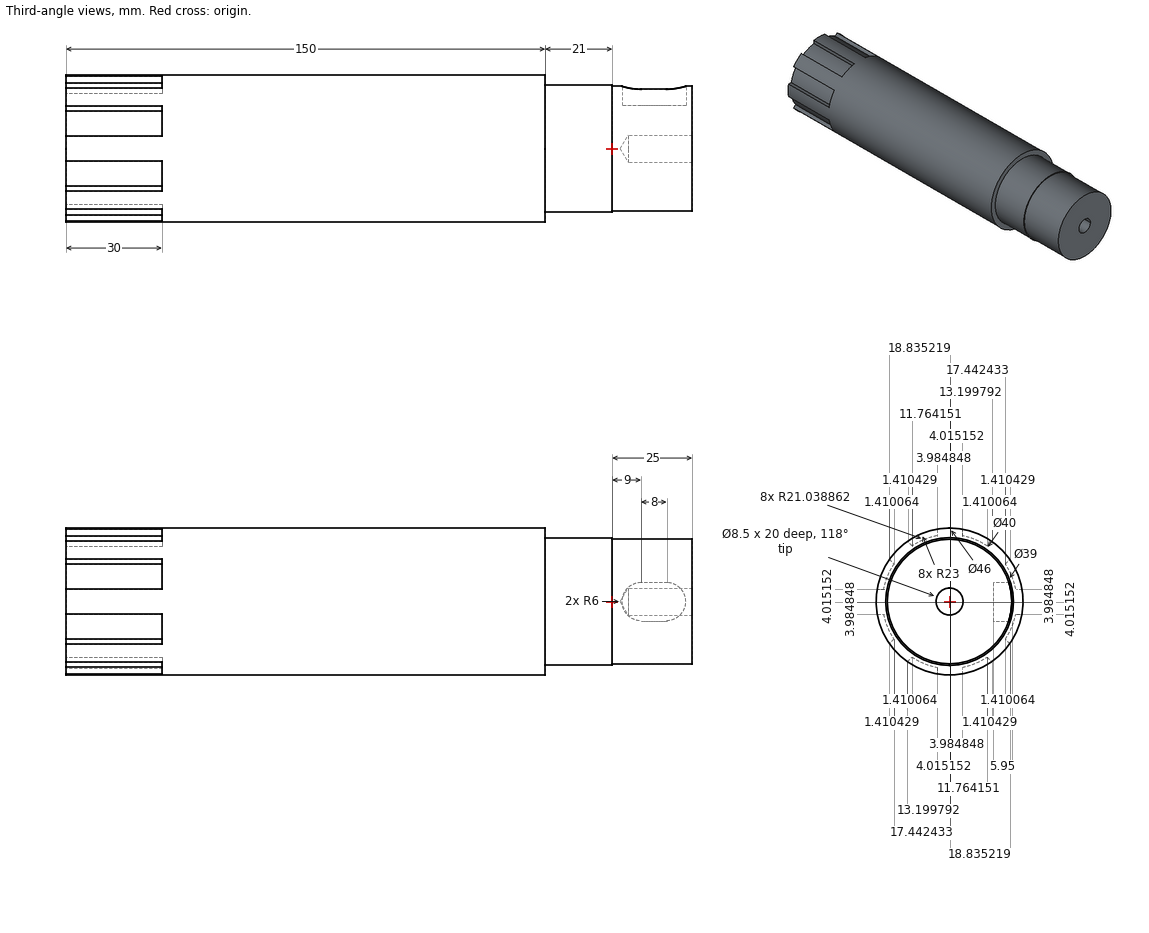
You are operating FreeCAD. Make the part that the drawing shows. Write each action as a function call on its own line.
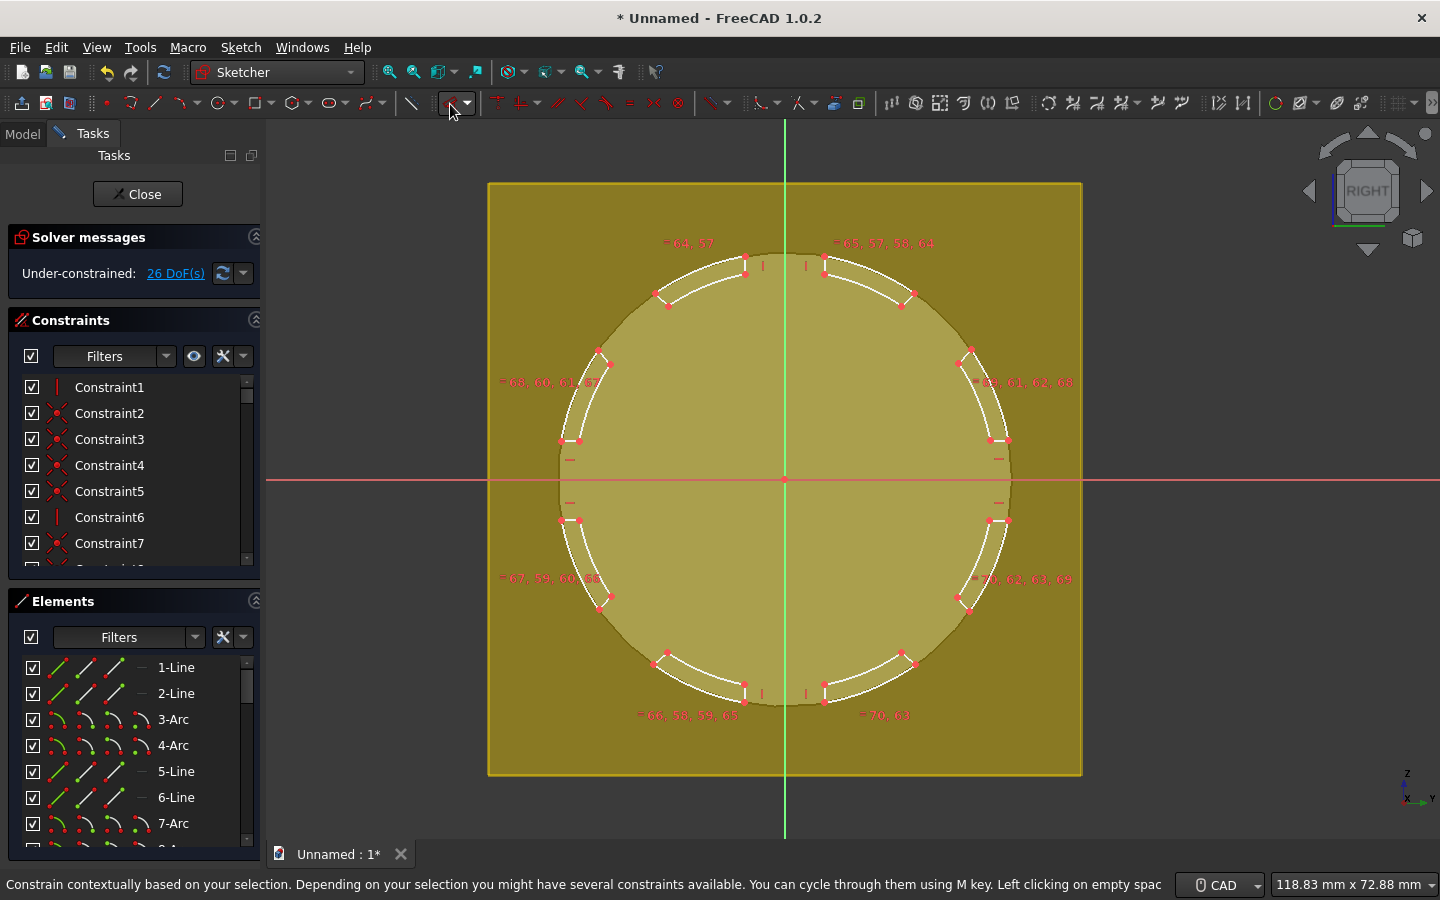
click(721, 280)
click(711, 250)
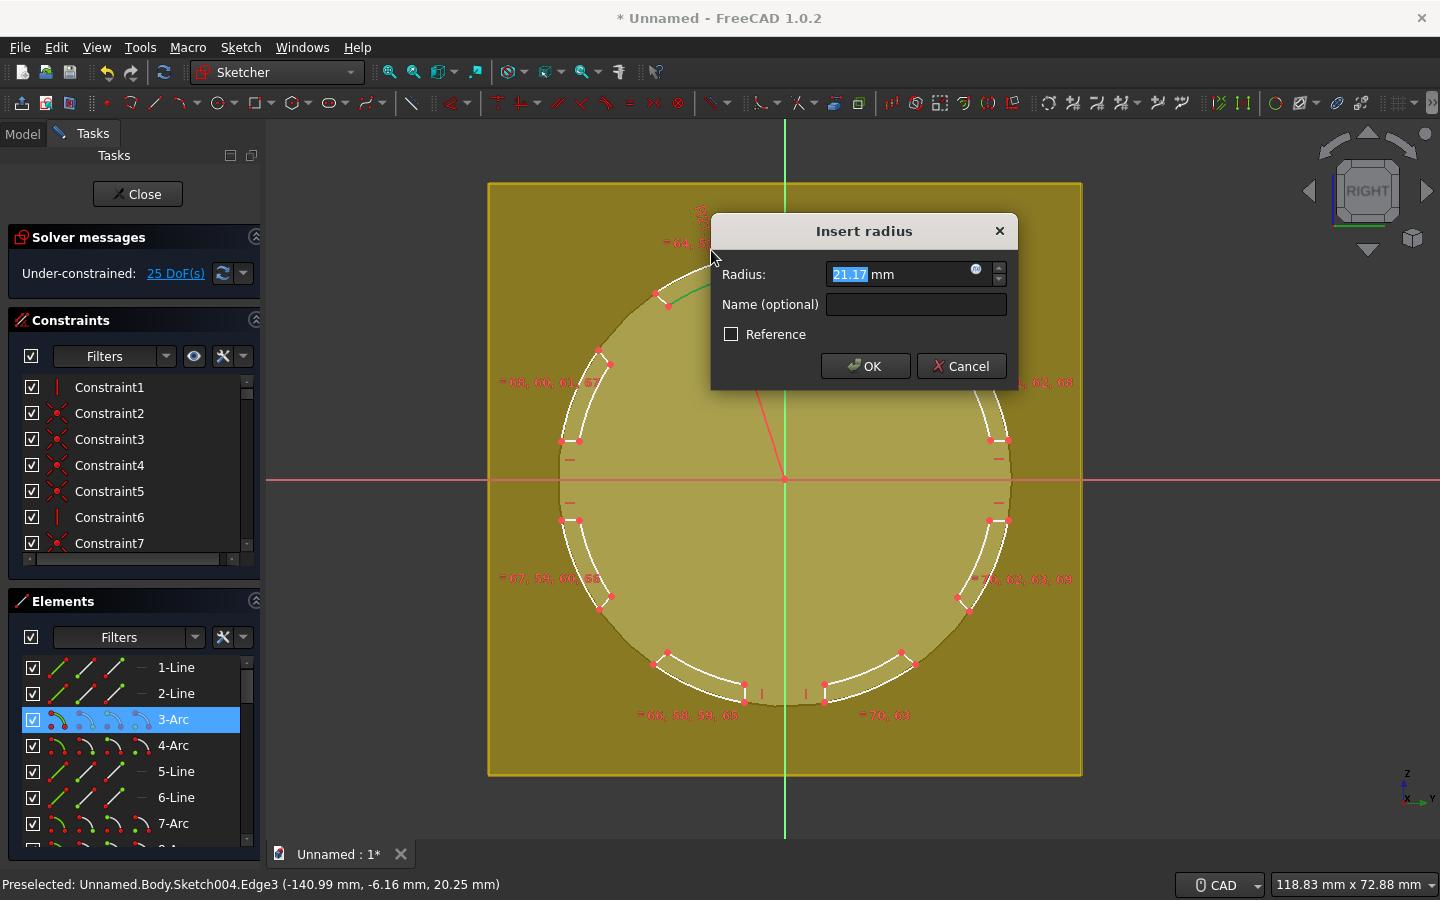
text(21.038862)
key(Return)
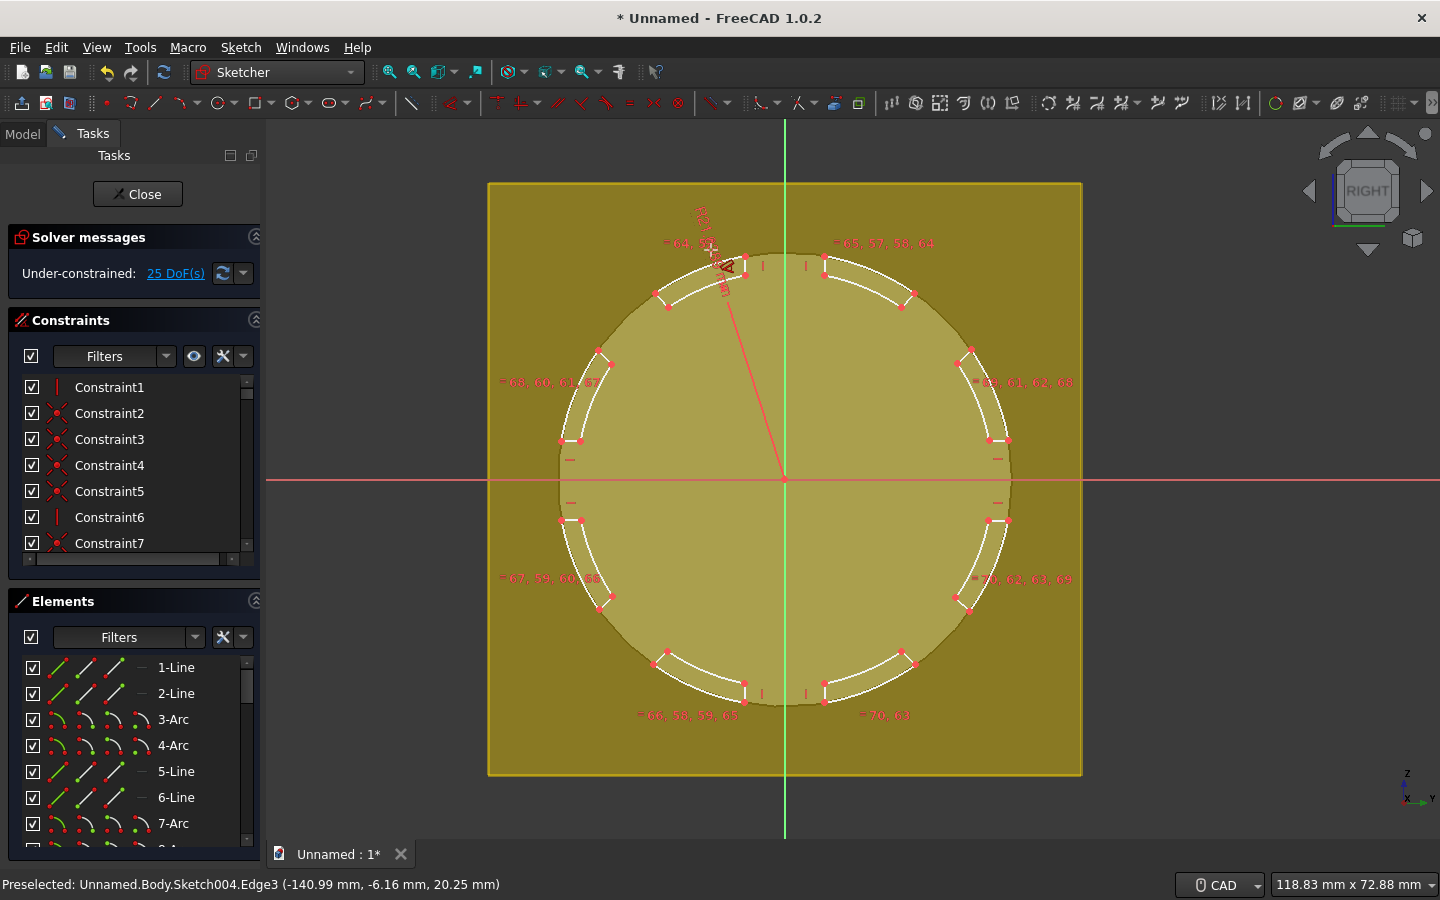
click(717, 263)
click(835, 226)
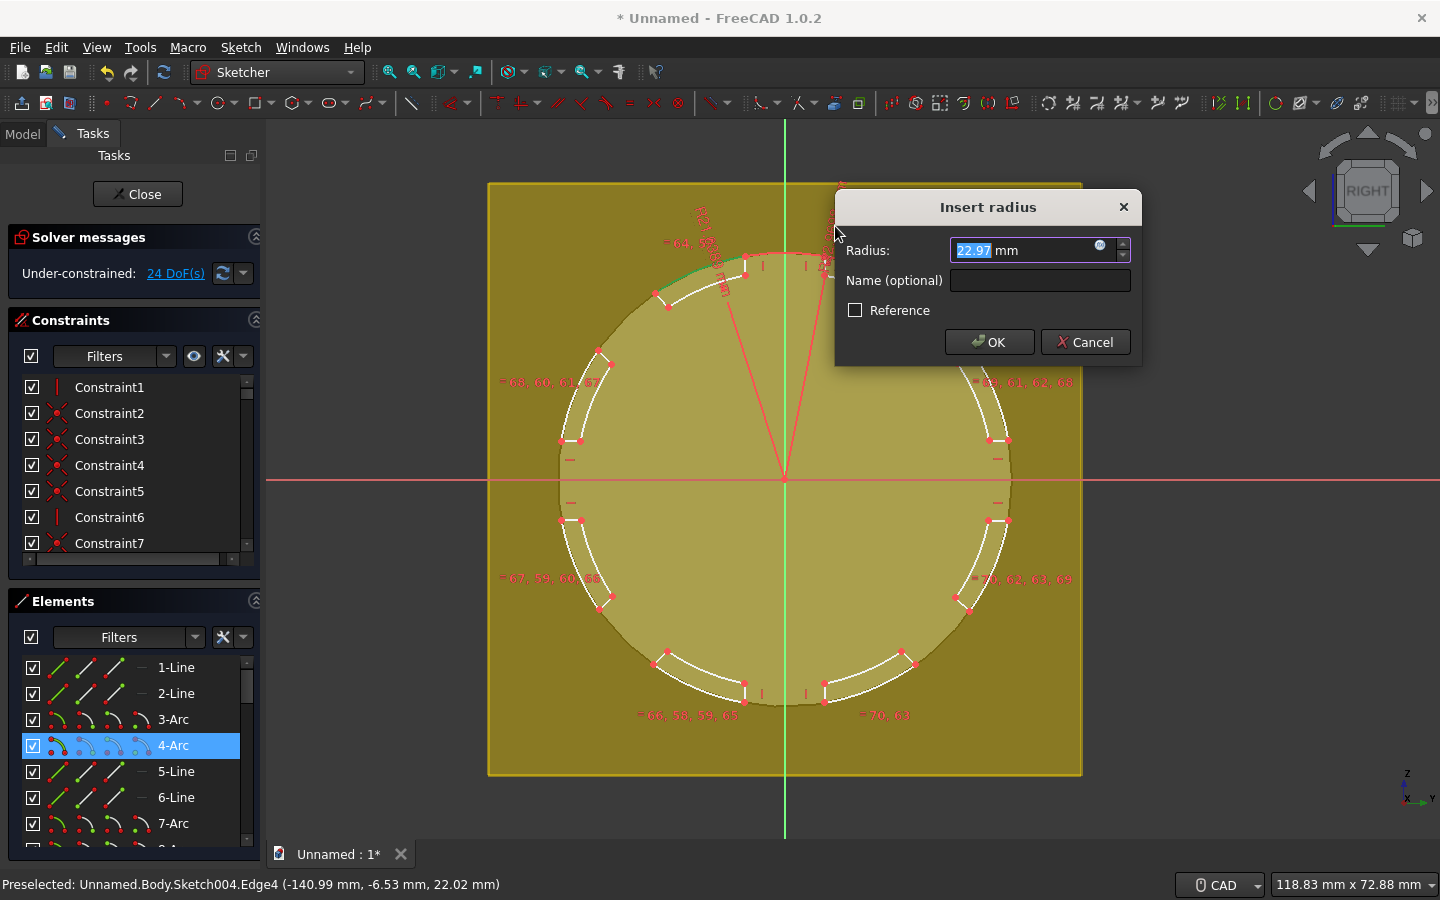
text(23)
key(Return)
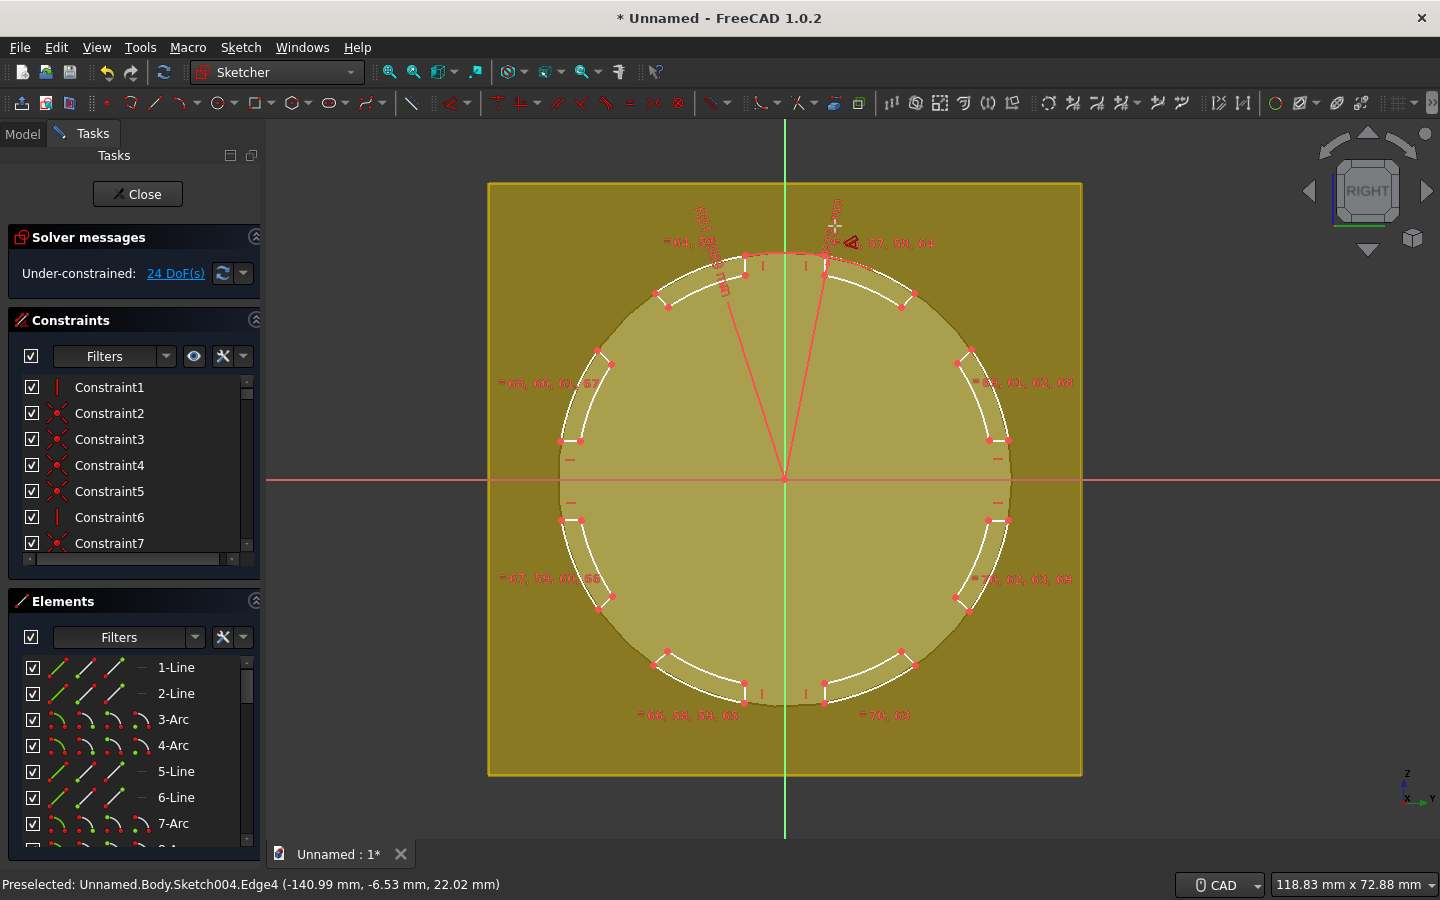
click(745, 256)
click(765, 222)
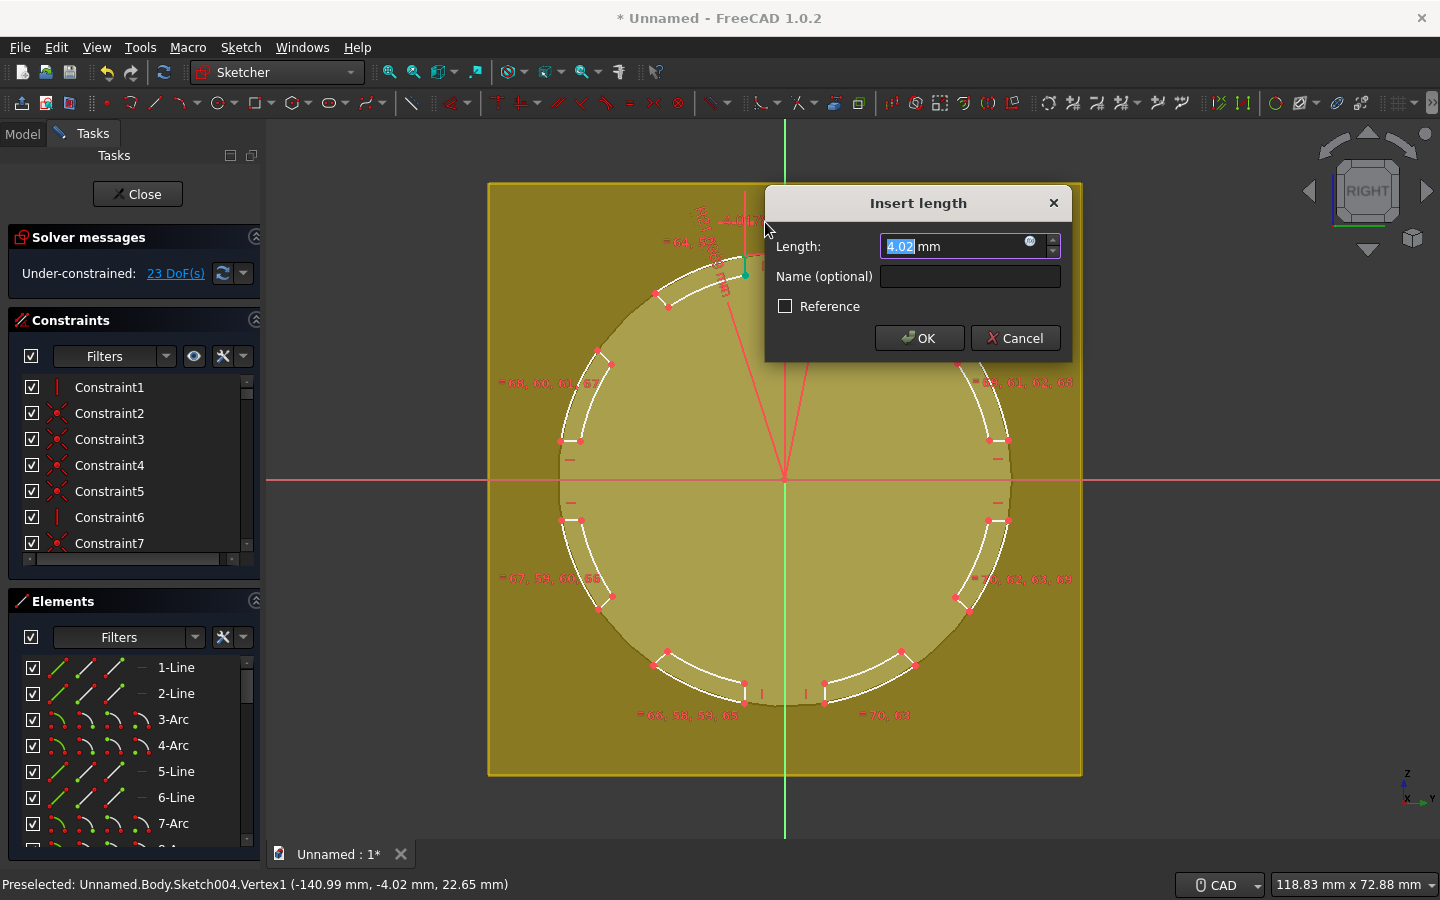
text(3.984848)
key(Return)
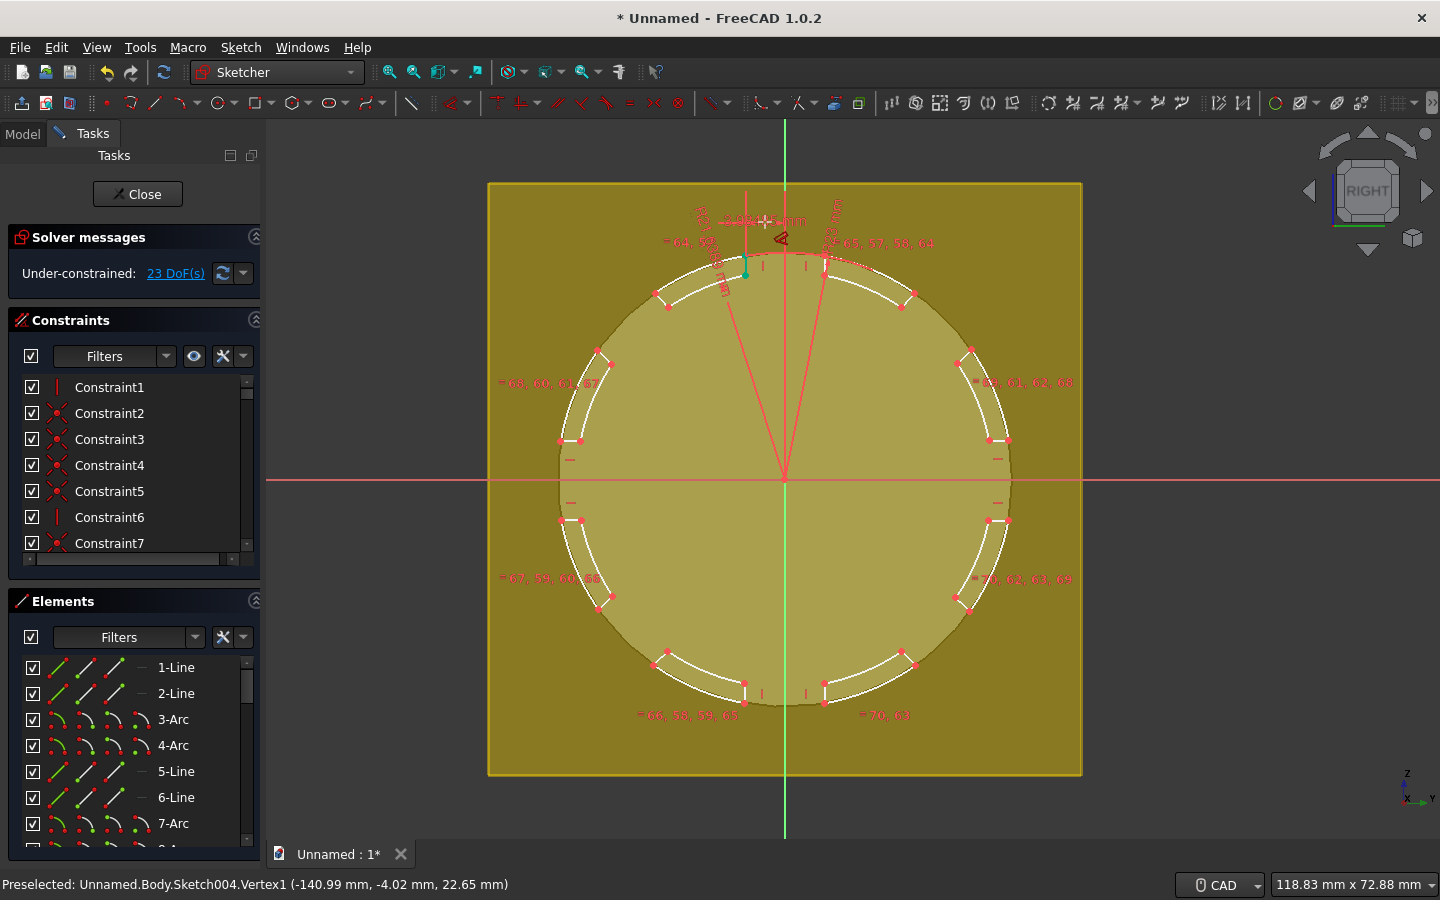
click(825, 276)
click(805, 514)